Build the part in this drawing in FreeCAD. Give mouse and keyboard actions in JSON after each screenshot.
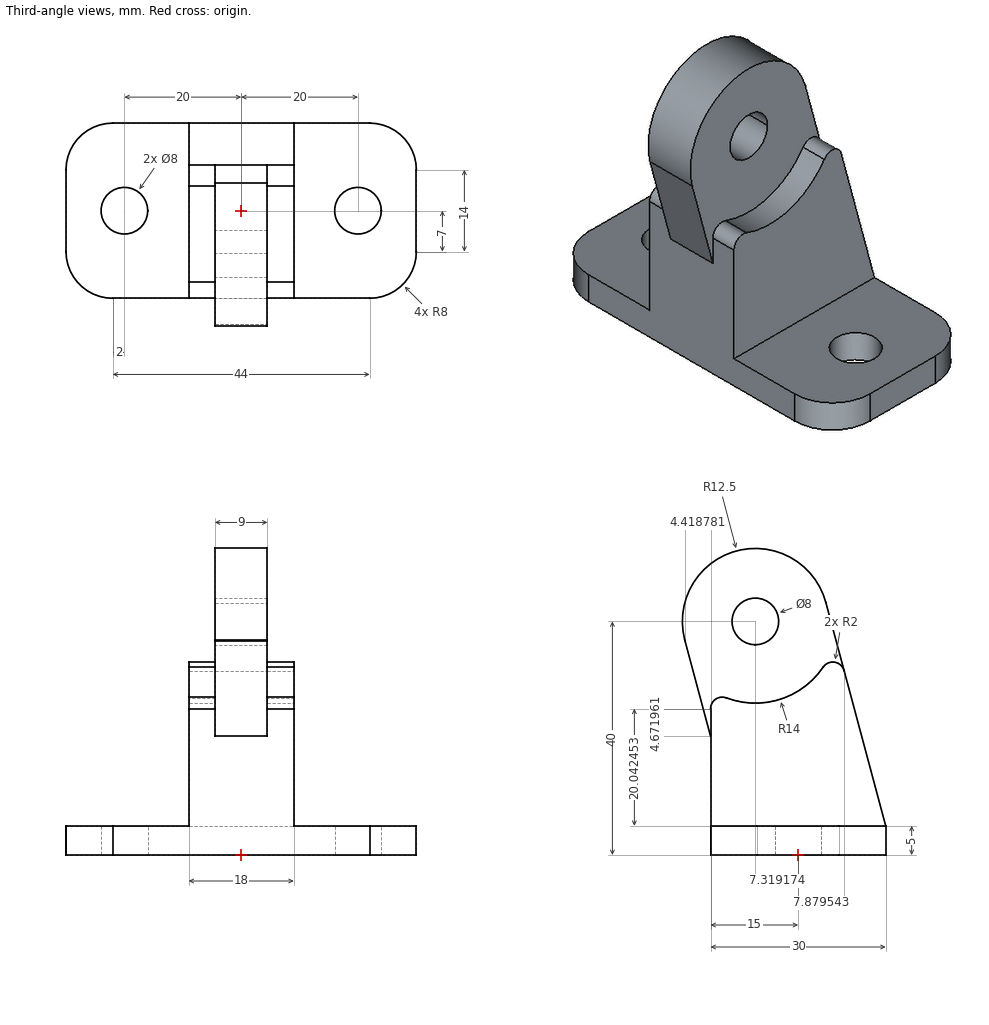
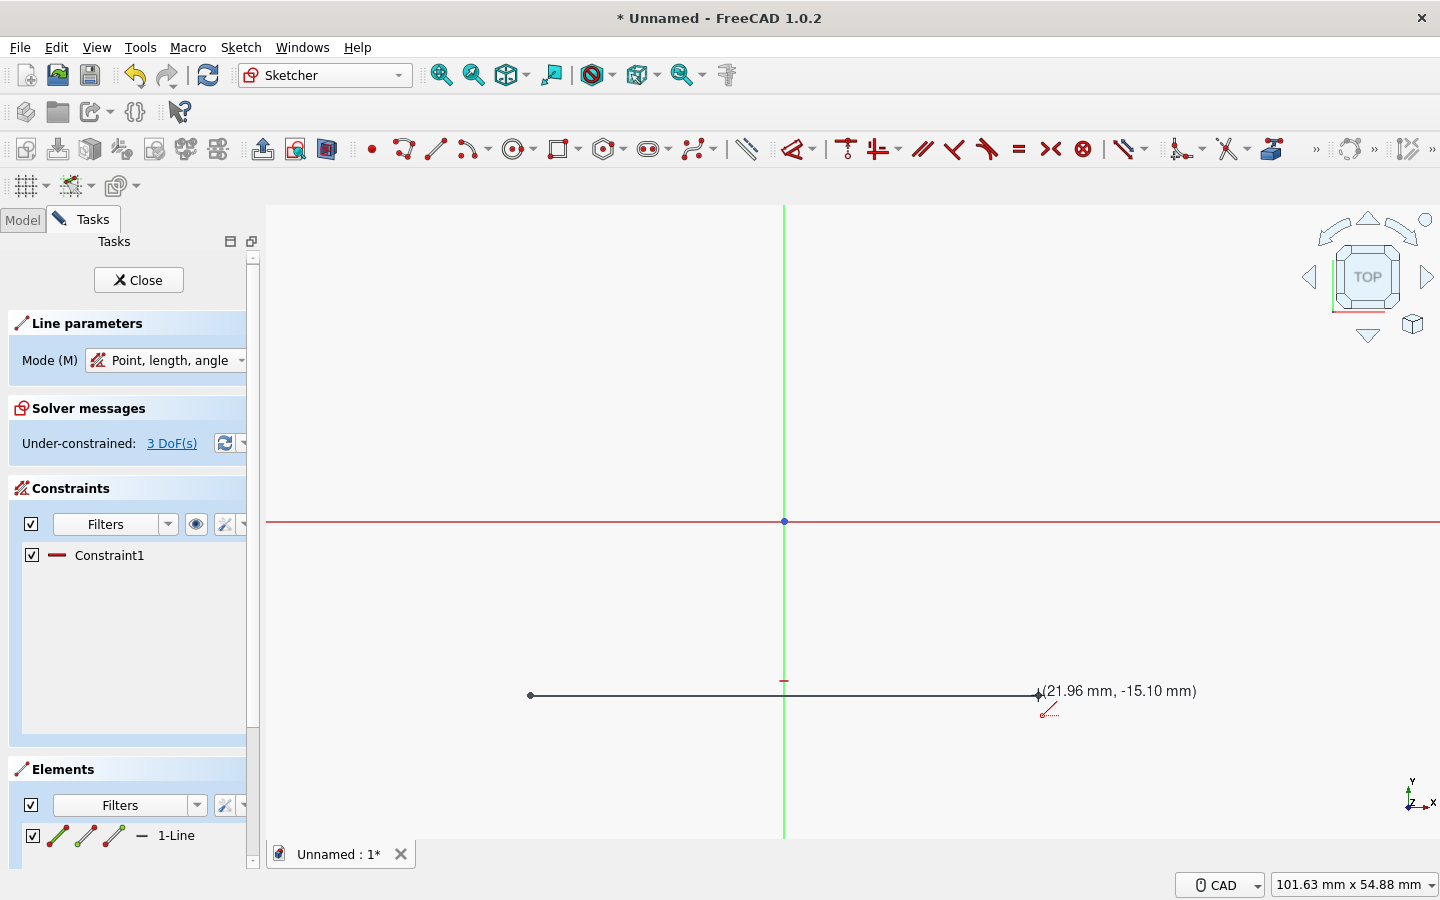
{"action": "left_click", "coordinate": [1131, 602]}
{"action": "left_click", "coordinate": [1131, 441]}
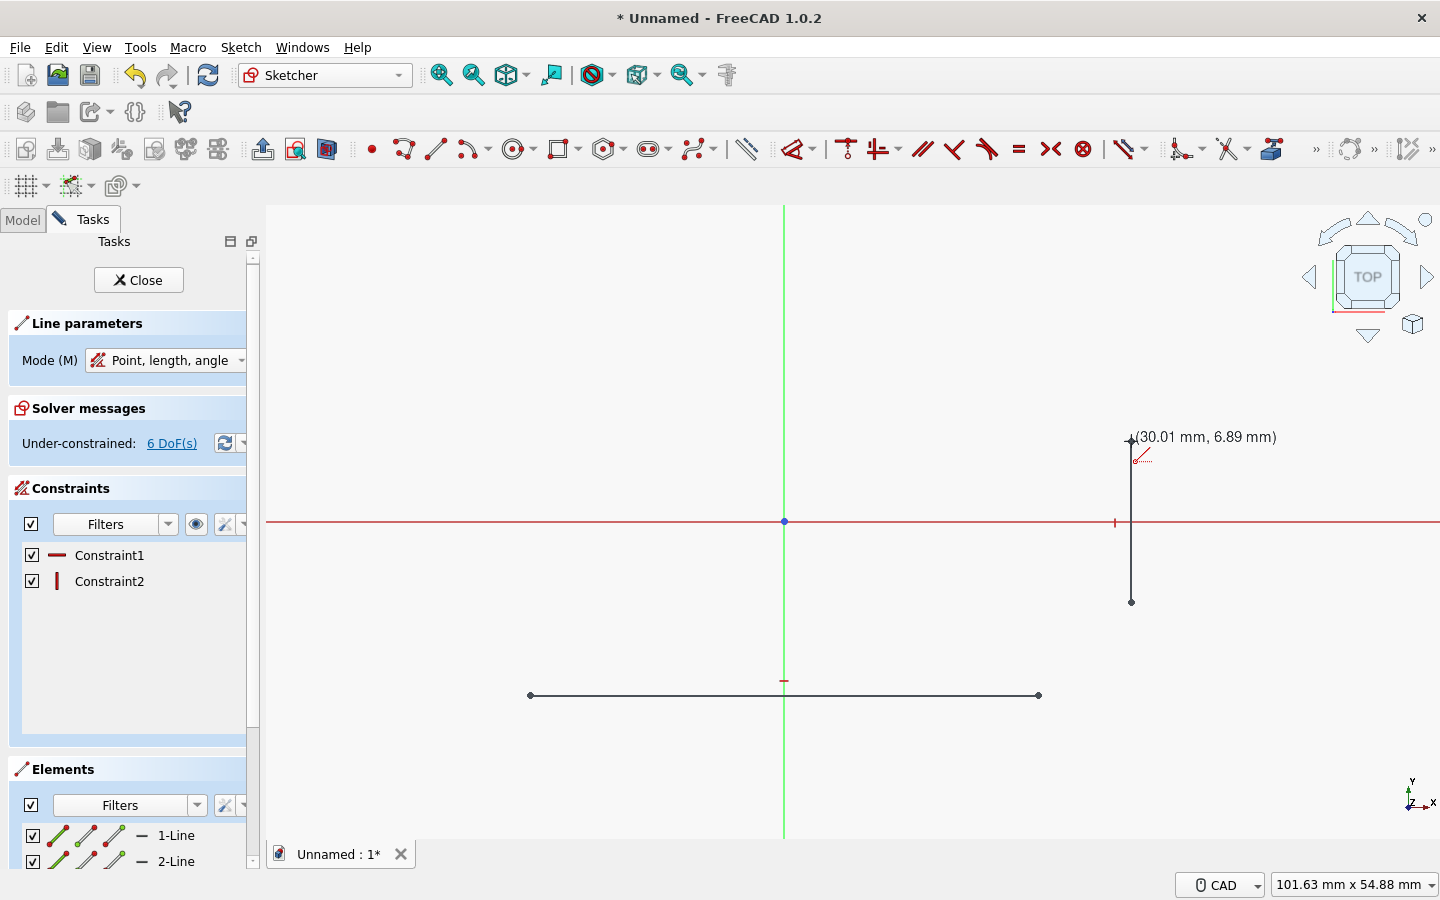
{"action": "left_click", "coordinate": [1038, 348]}
{"action": "left_click", "coordinate": [530, 348]}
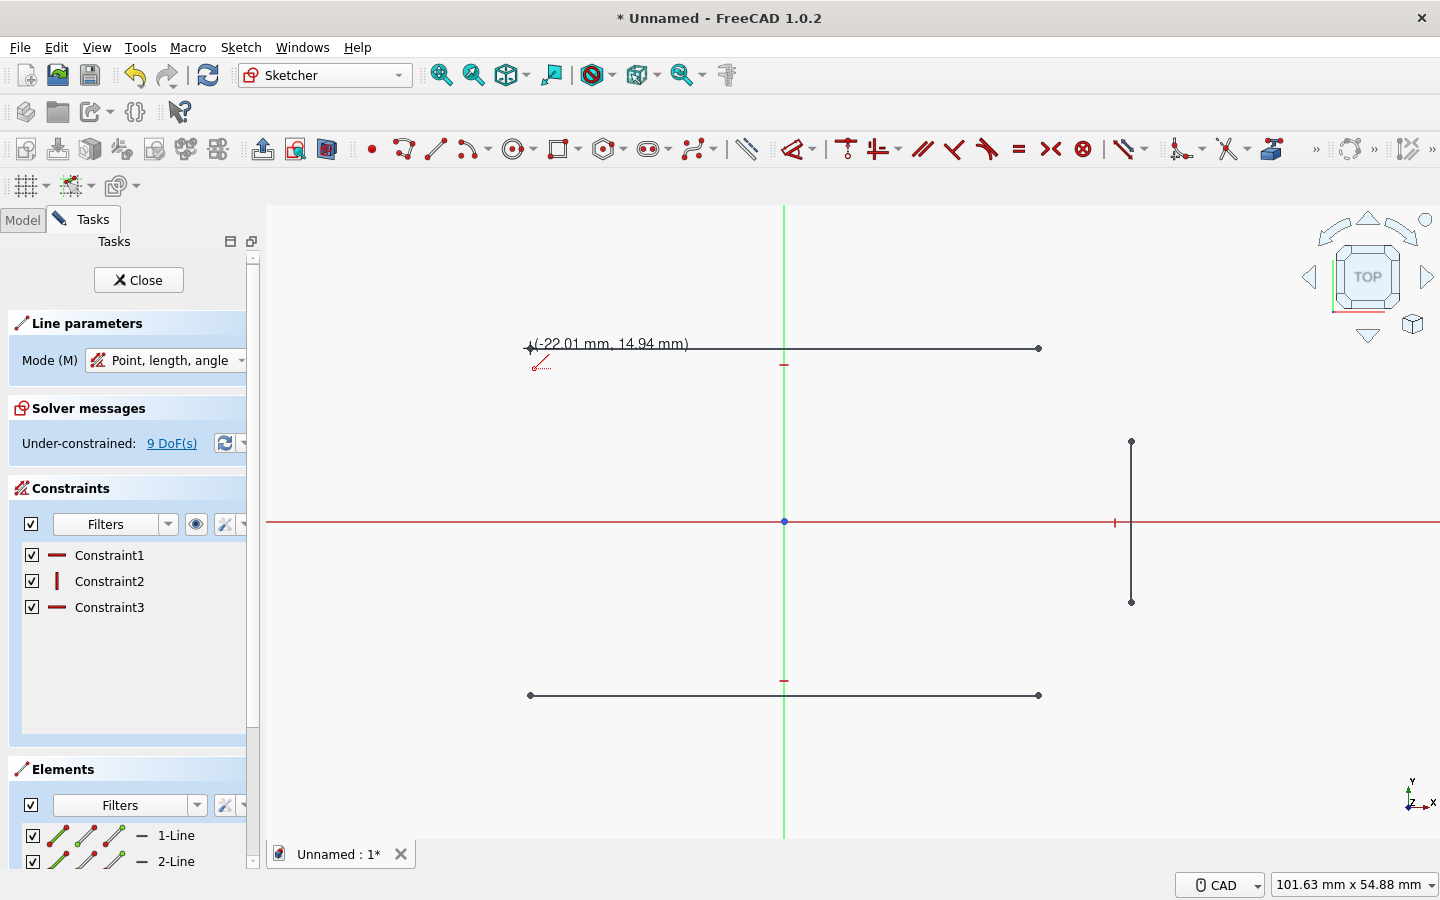
{"action": "left_click", "coordinate": [438, 441]}
{"action": "left_click", "coordinate": [438, 602]}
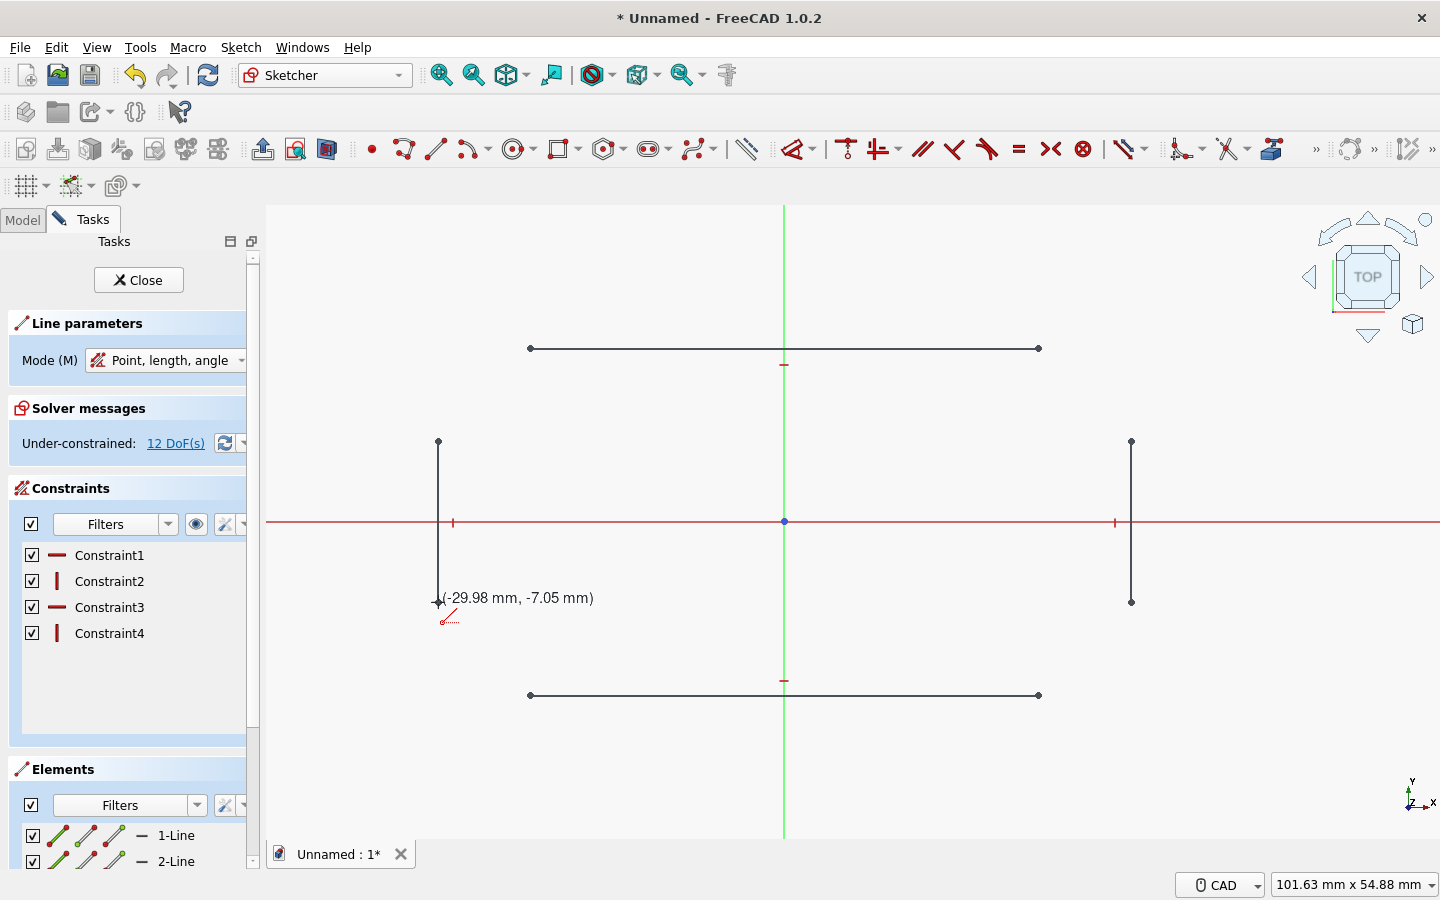
{"action": "key", "text": "g 3 a"}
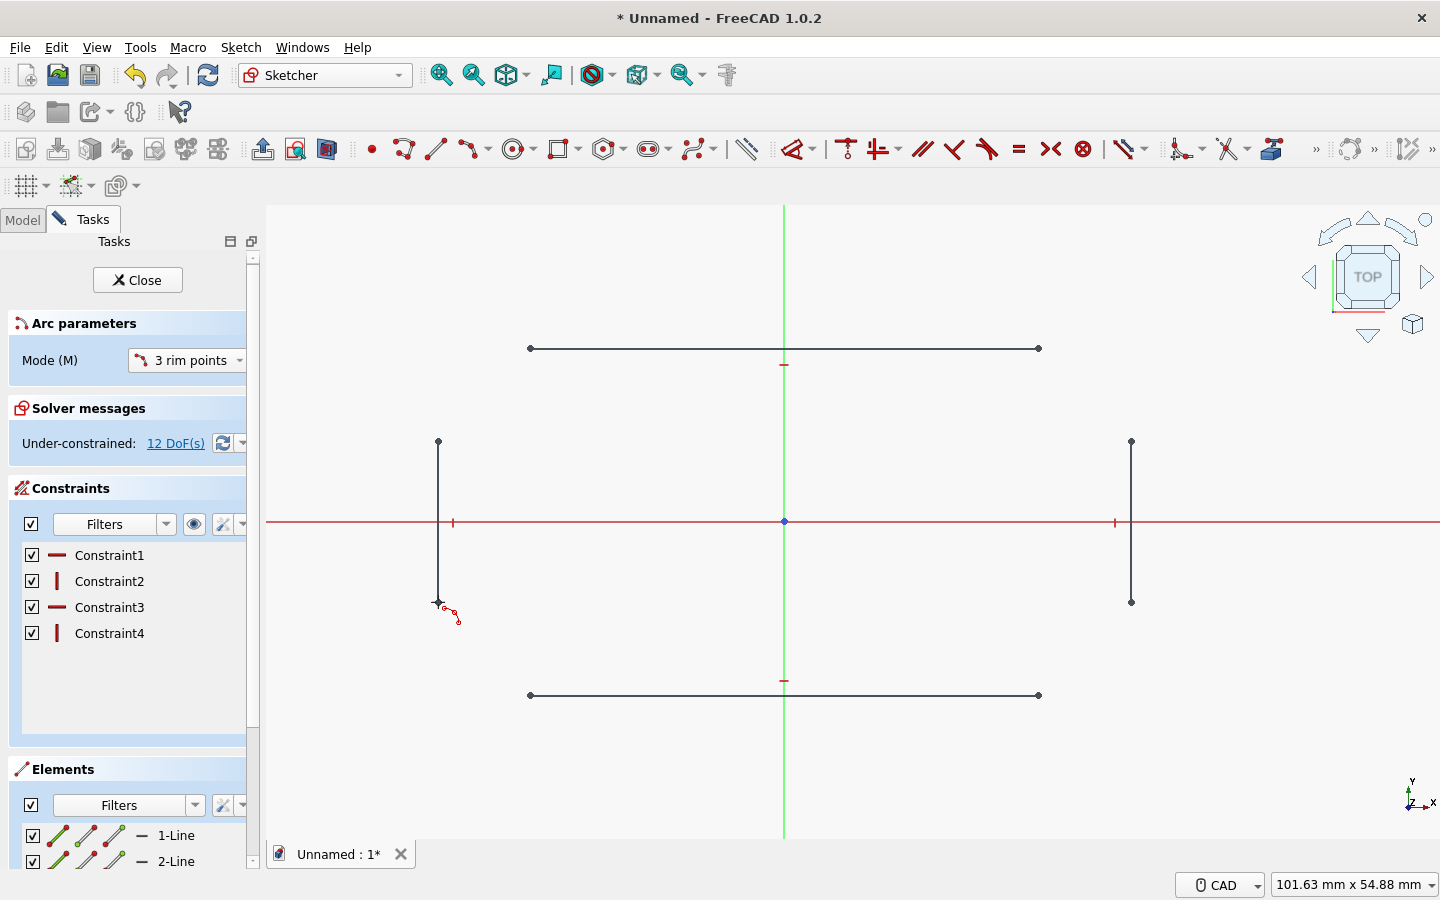
{"action": "left_click", "coordinate": [1038, 696]}
{"action": "left_click", "coordinate": [1131, 603]}
{"action": "left_click", "coordinate": [1104, 668]}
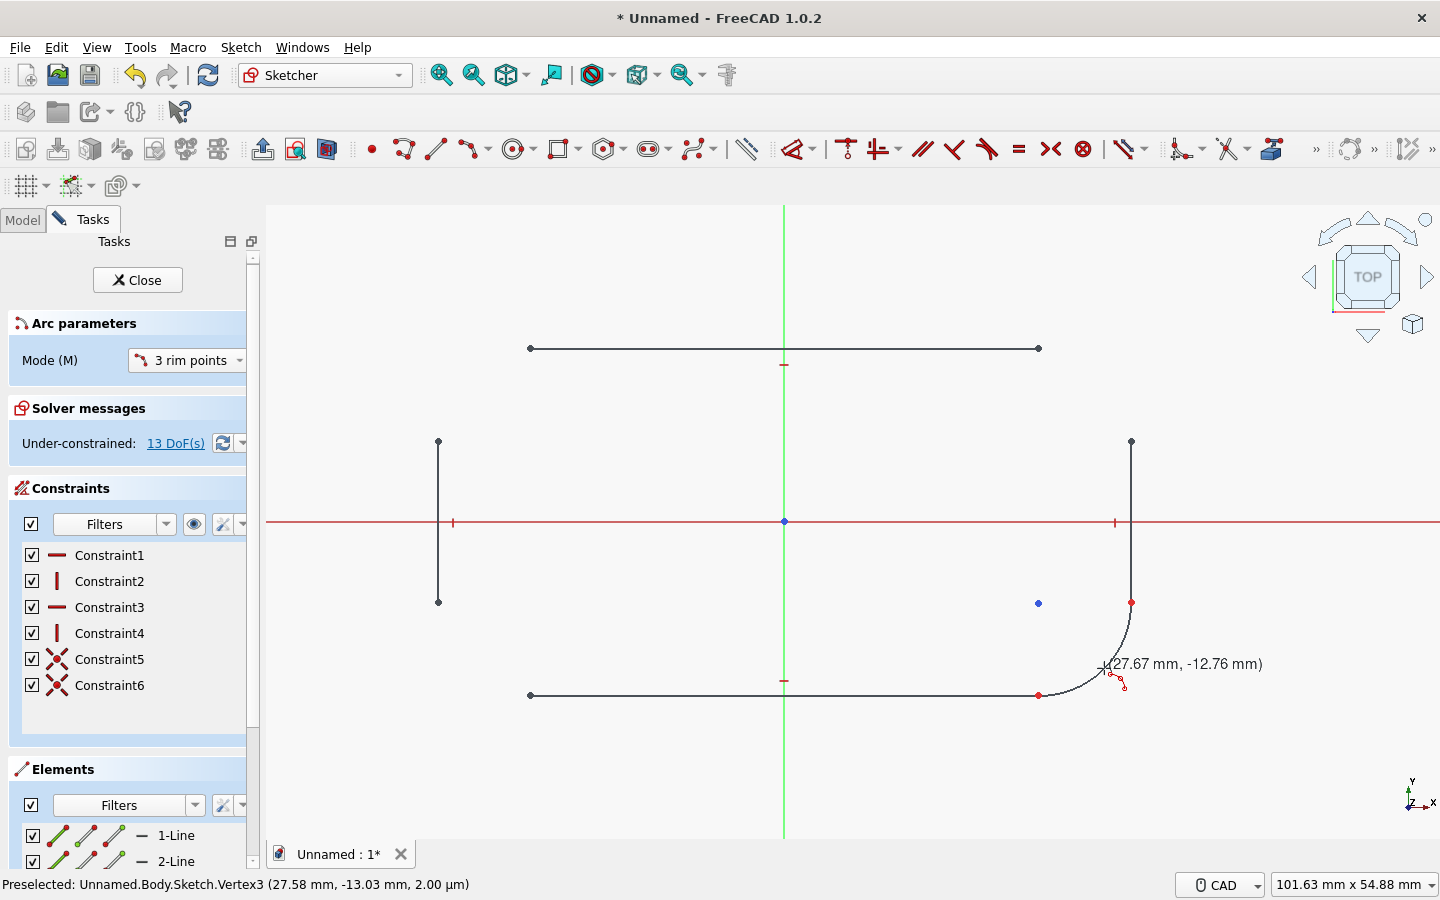
{"action": "left_click", "coordinate": [1131, 442]}
{"action": "left_click", "coordinate": [1038, 349]}
{"action": "left_click", "coordinate": [1104, 375]}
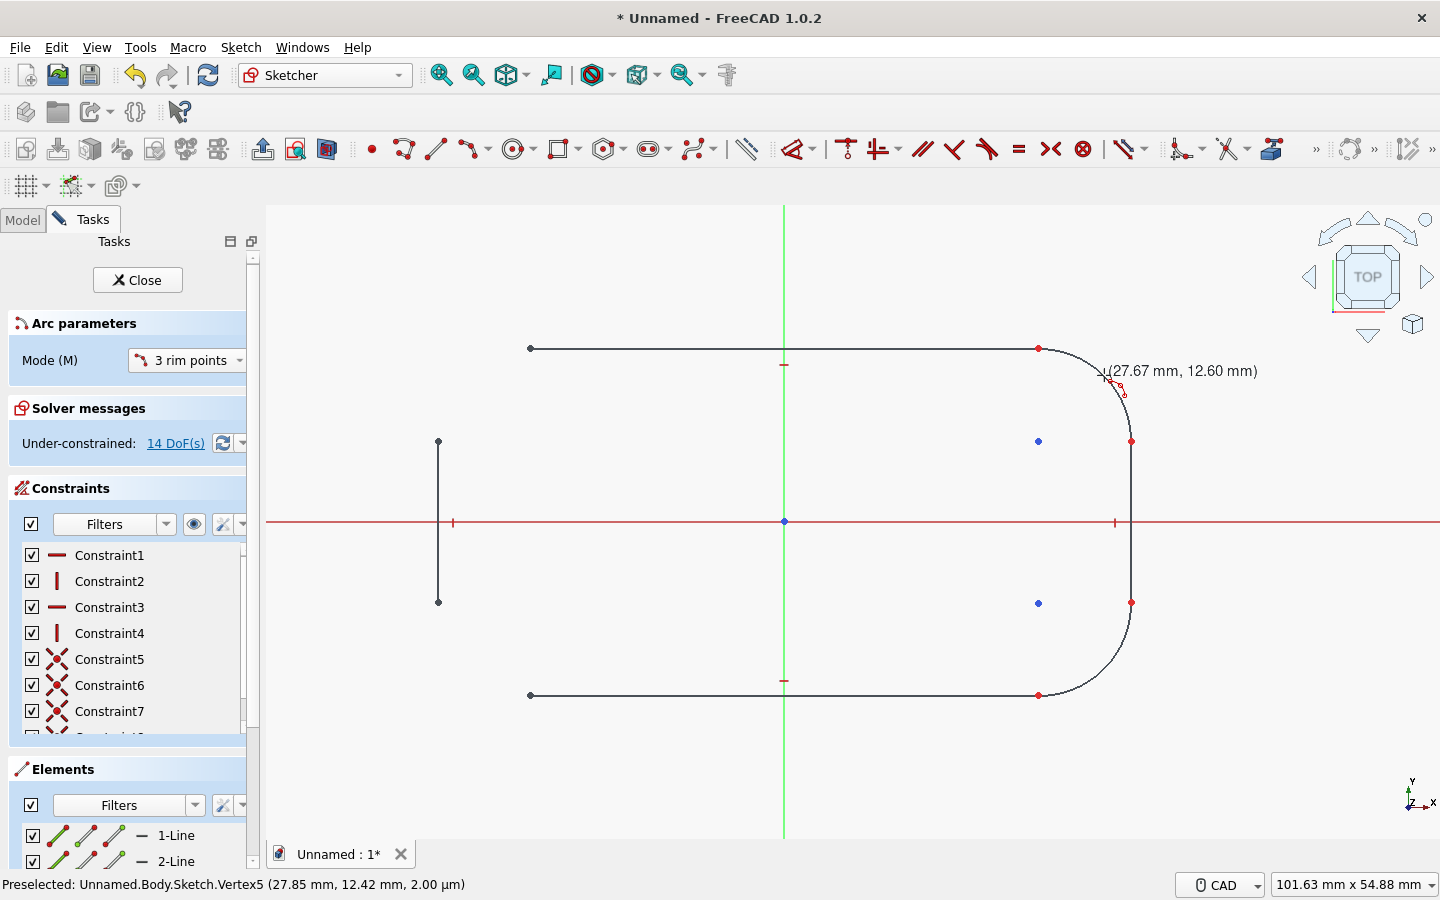
{"action": "left_click", "coordinate": [530, 349]}
{"action": "left_click", "coordinate": [438, 442]}
{"action": "left_click", "coordinate": [465, 375]}